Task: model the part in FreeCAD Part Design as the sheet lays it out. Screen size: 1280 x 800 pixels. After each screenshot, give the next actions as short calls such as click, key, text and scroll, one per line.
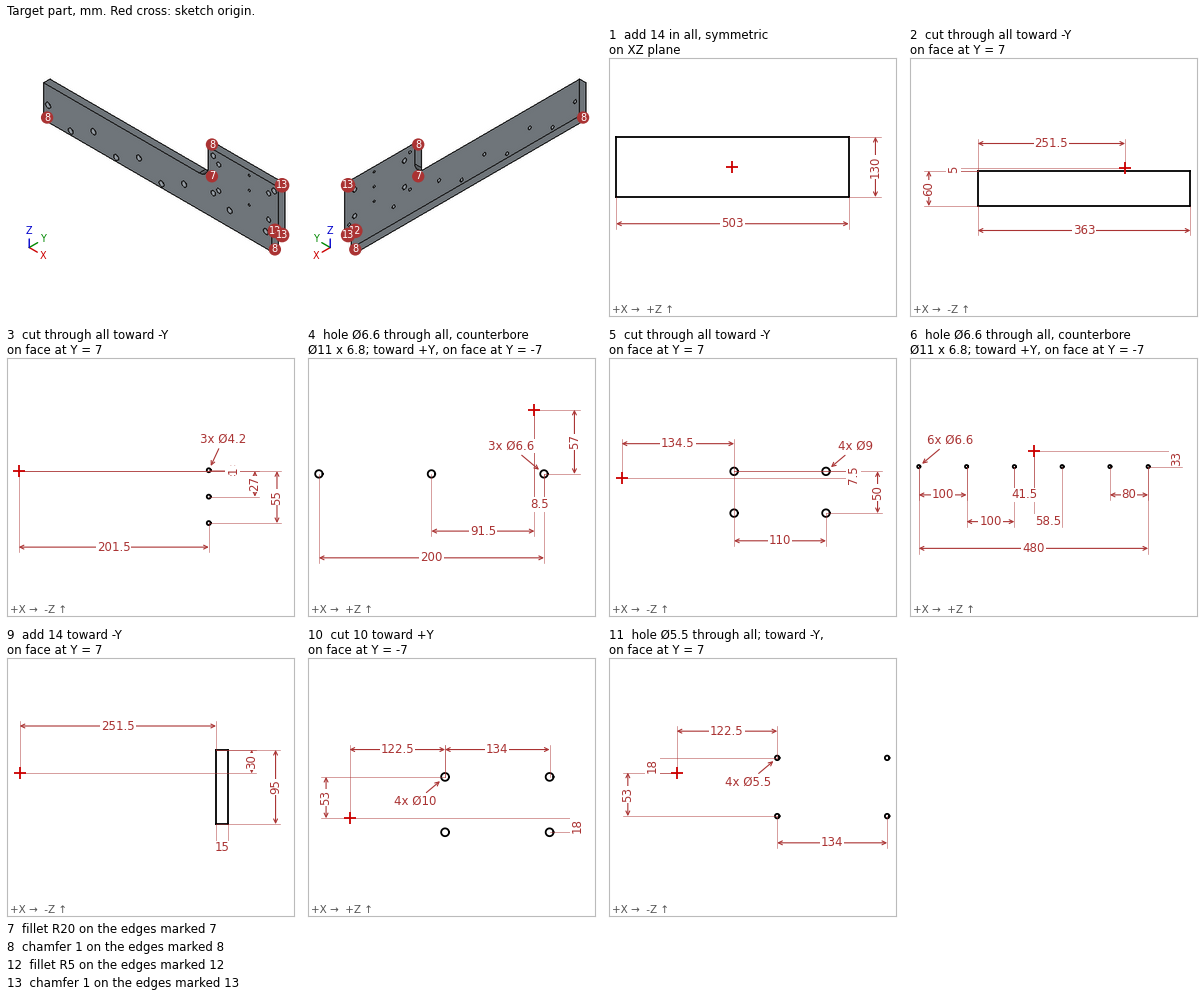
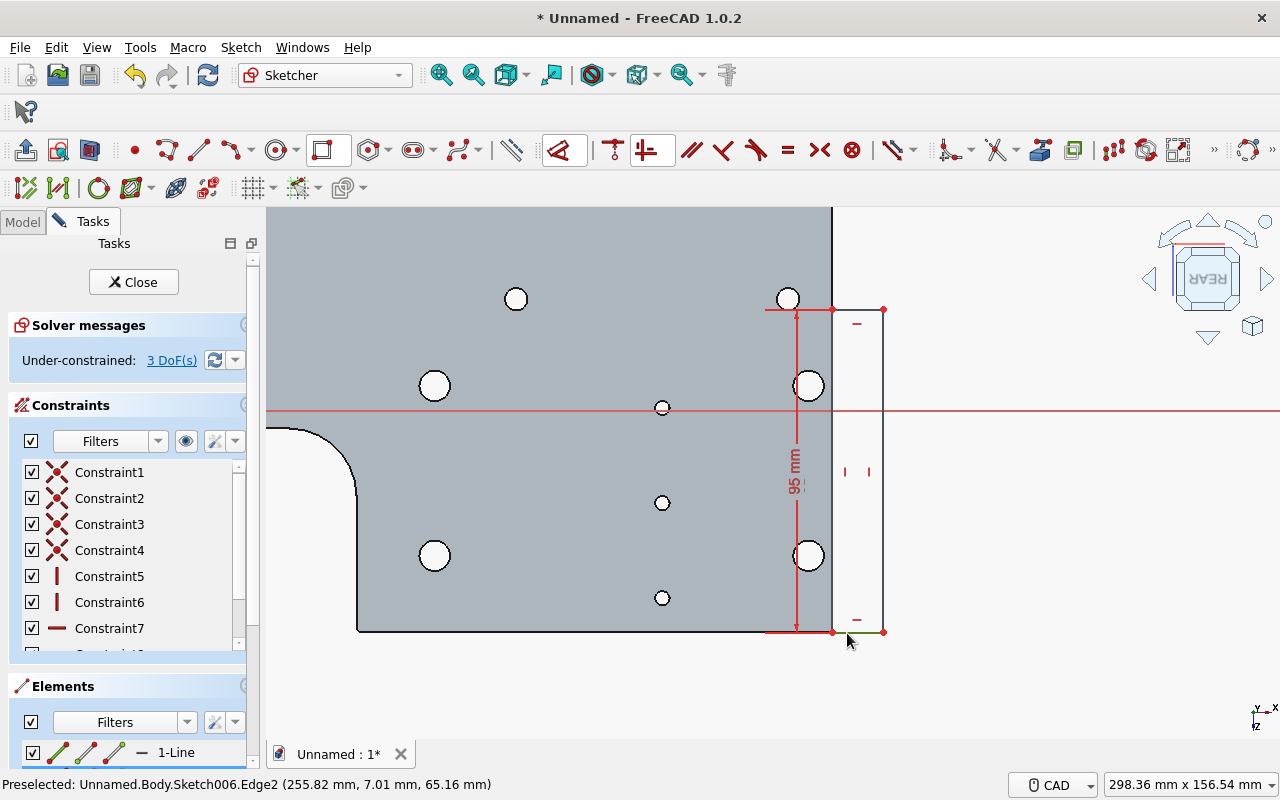
key(l)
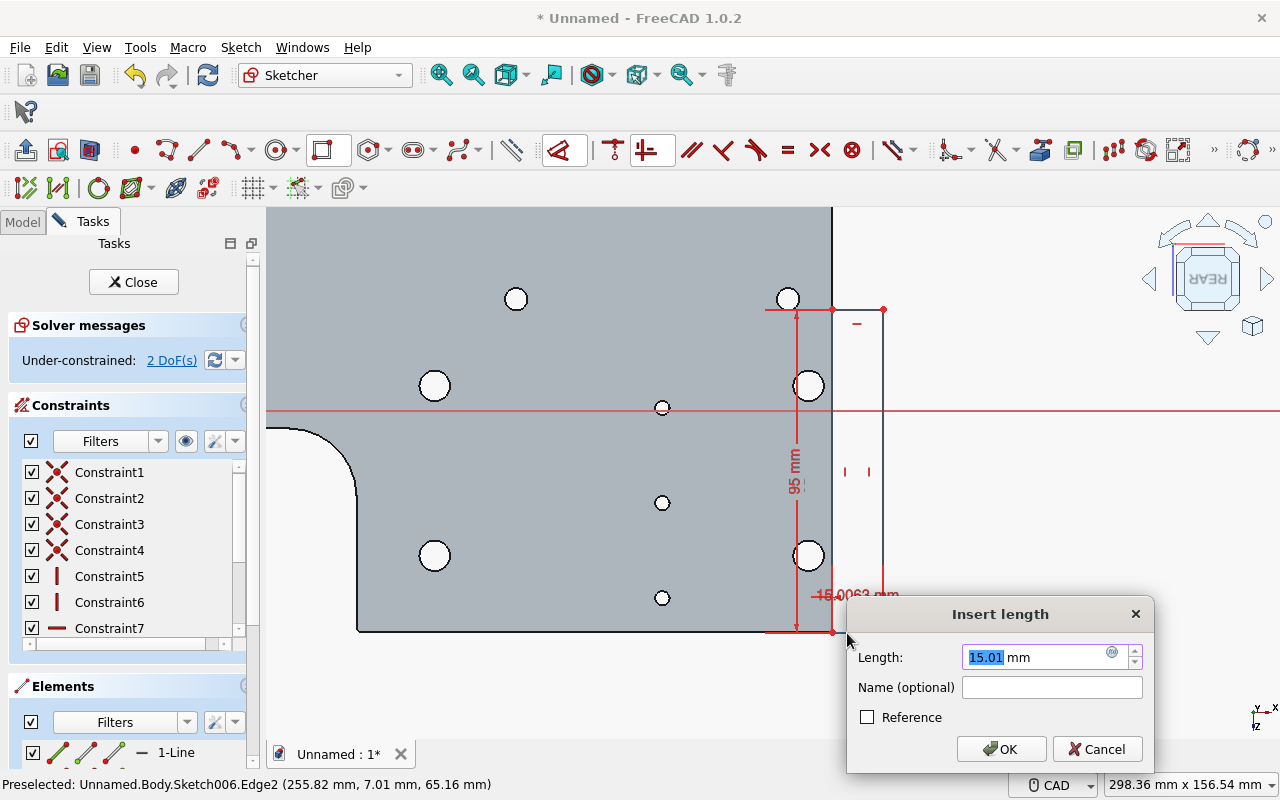
text(15)
key(Return)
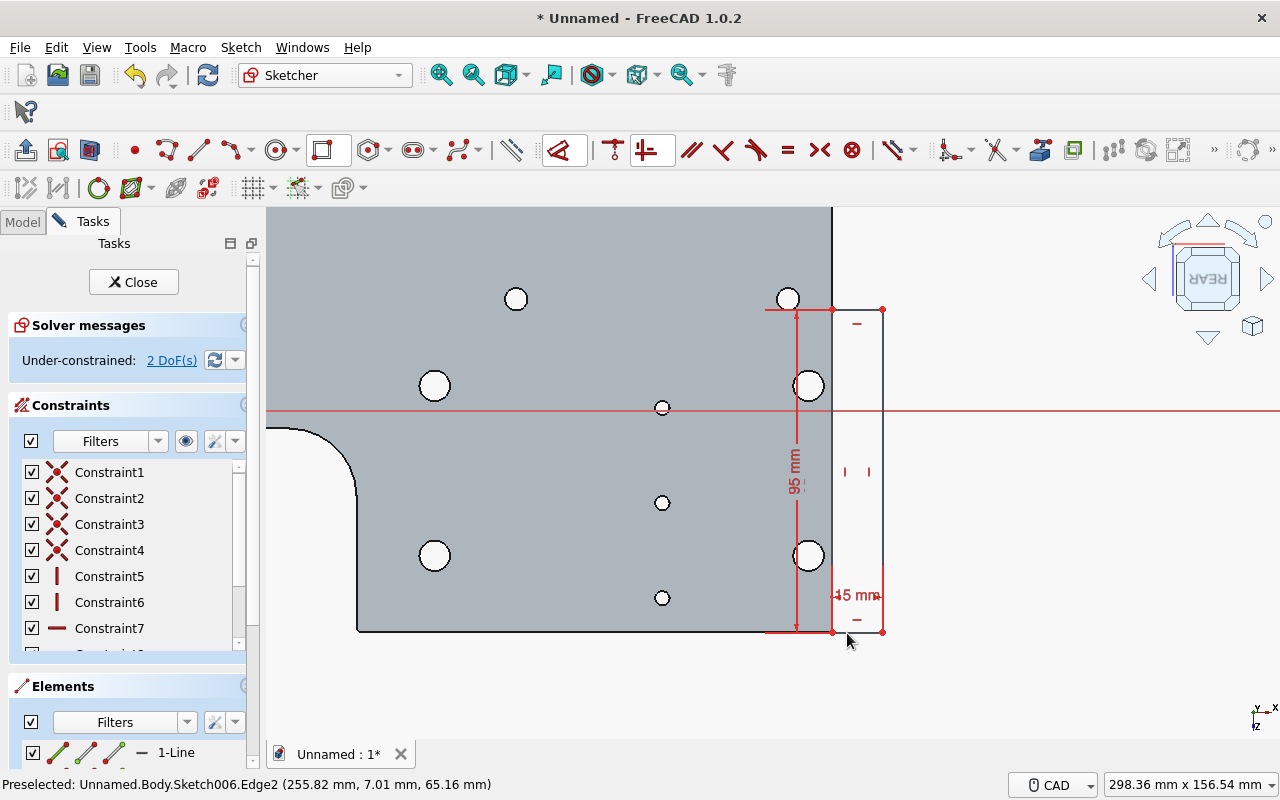
click(832, 310)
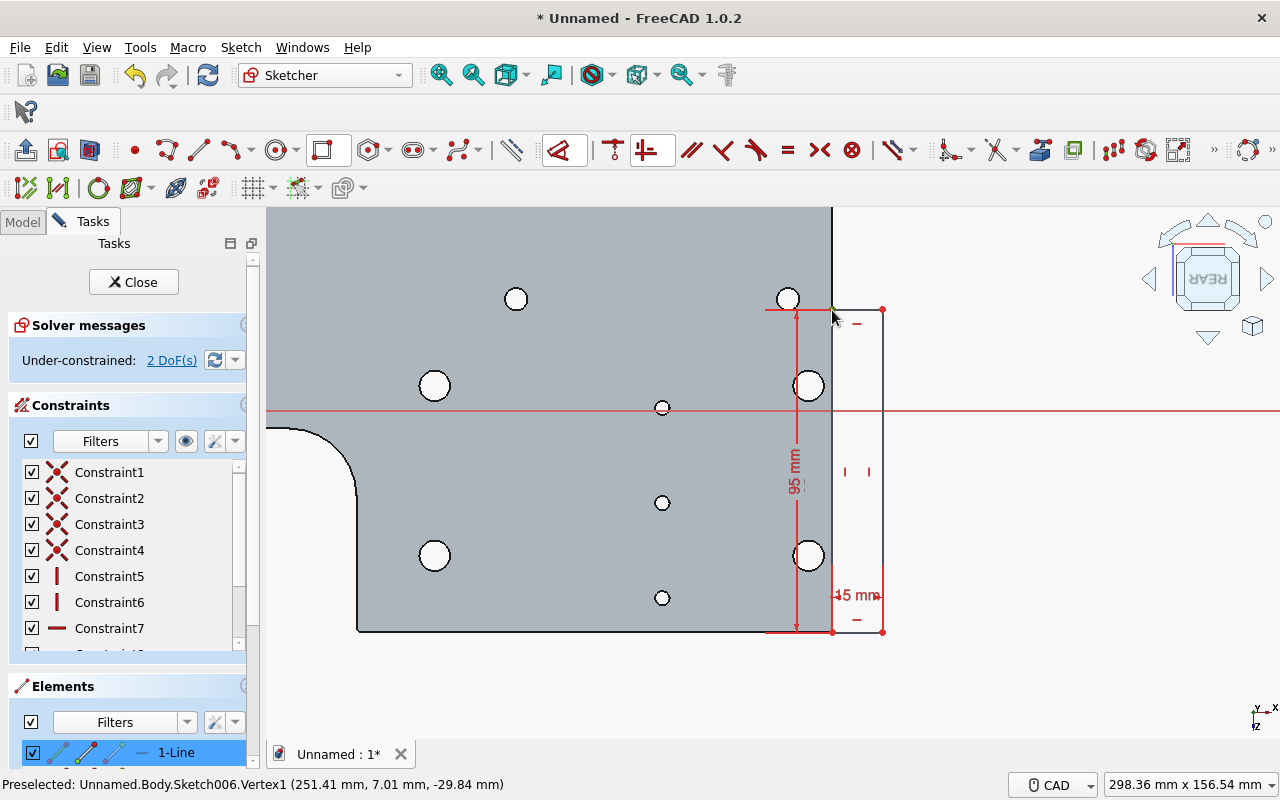
click(582, 150)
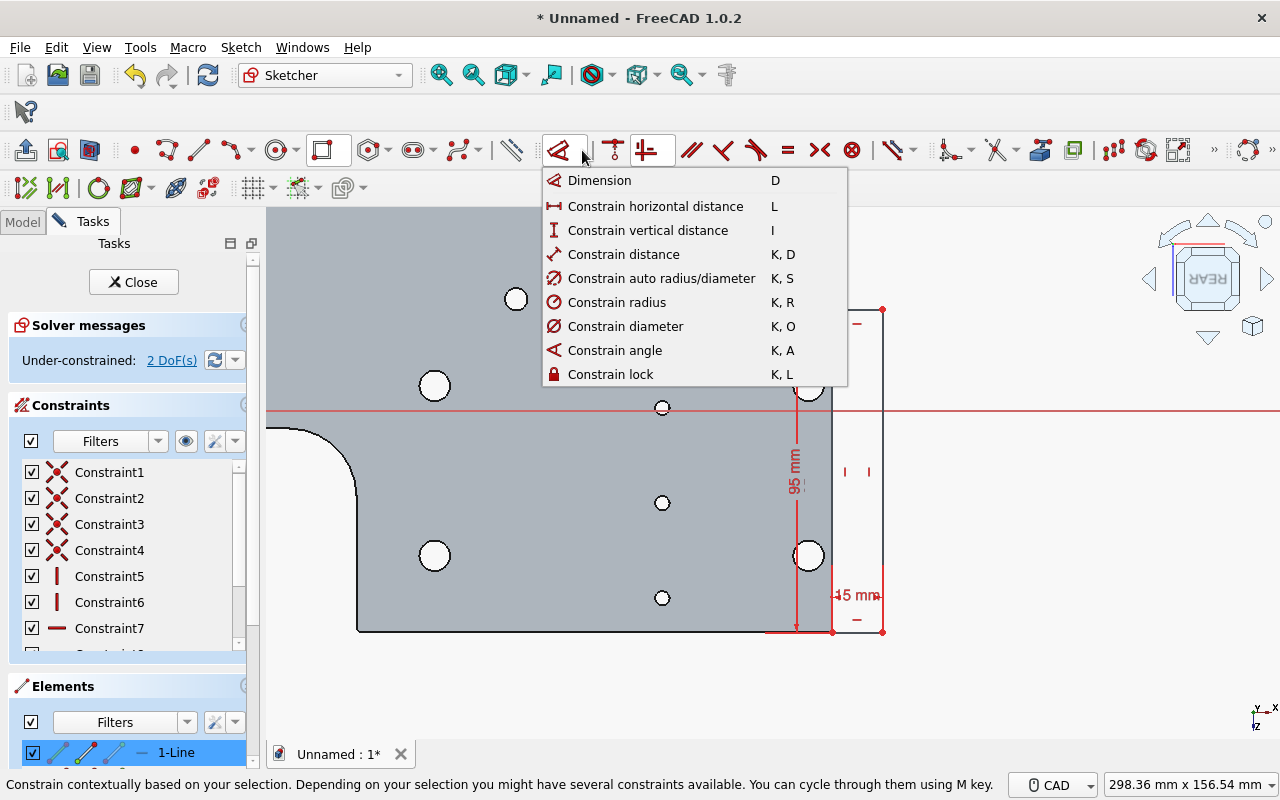
click(695, 230)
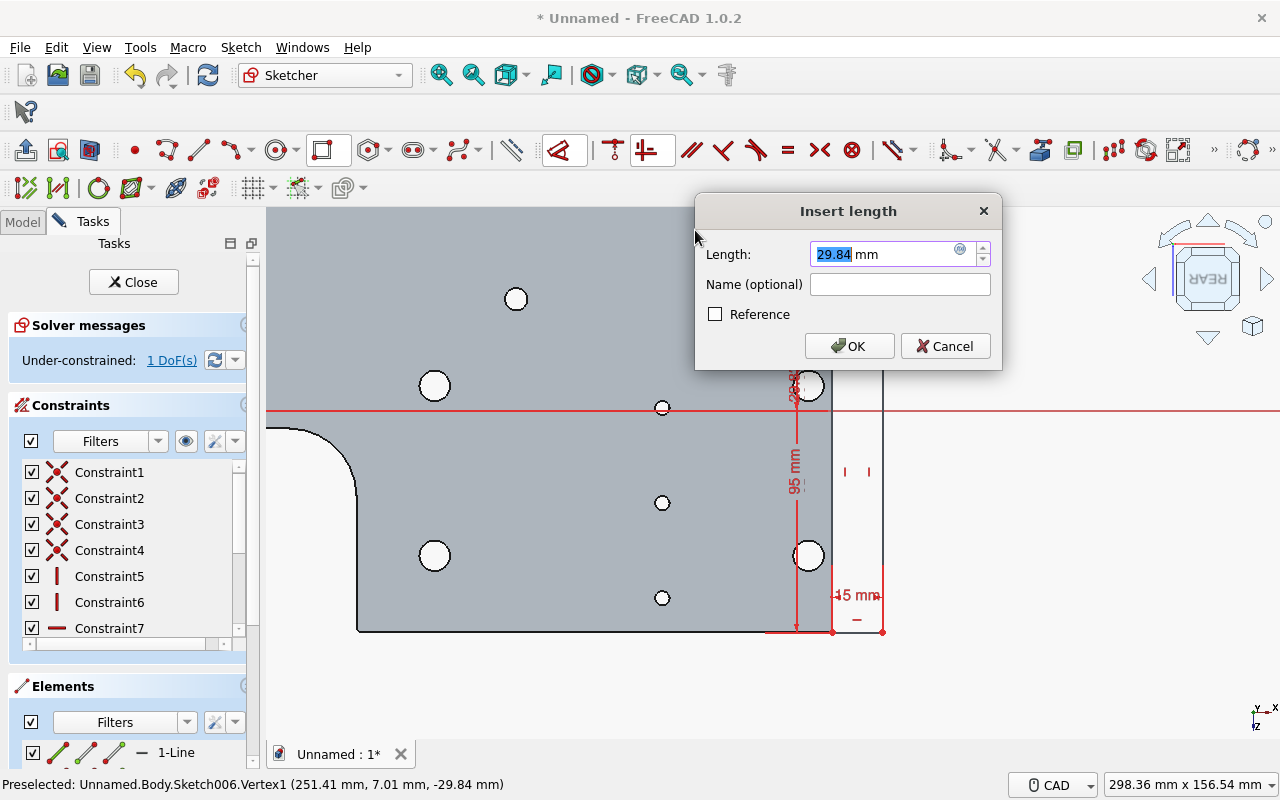
text(30)
key(Return)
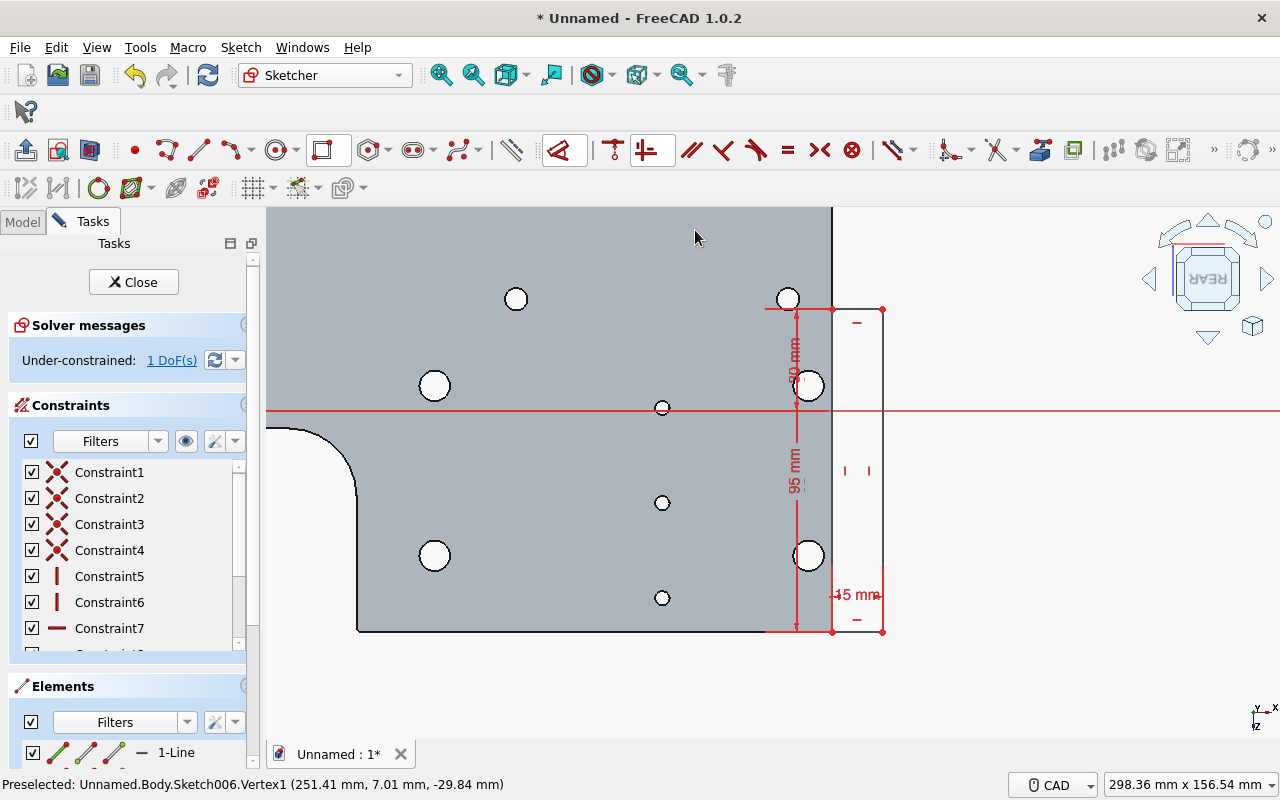
click(832, 309)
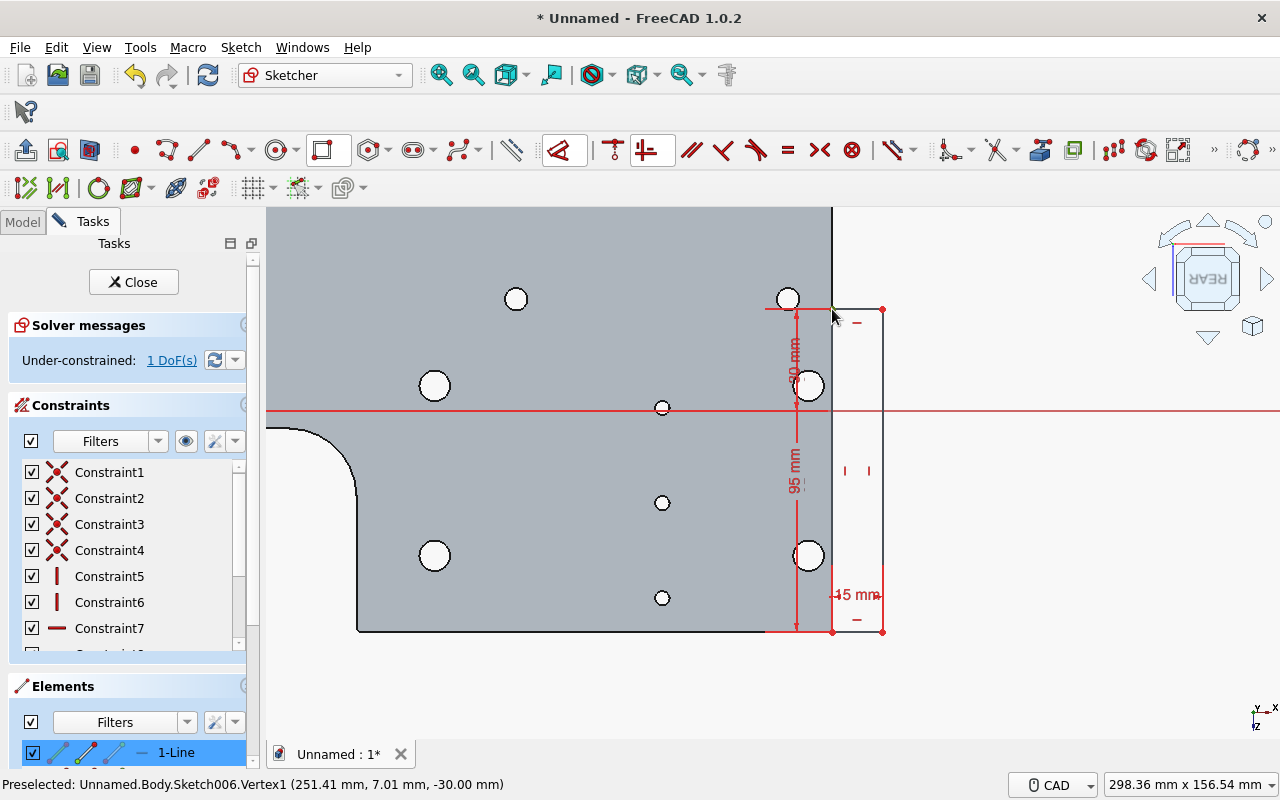
key(l)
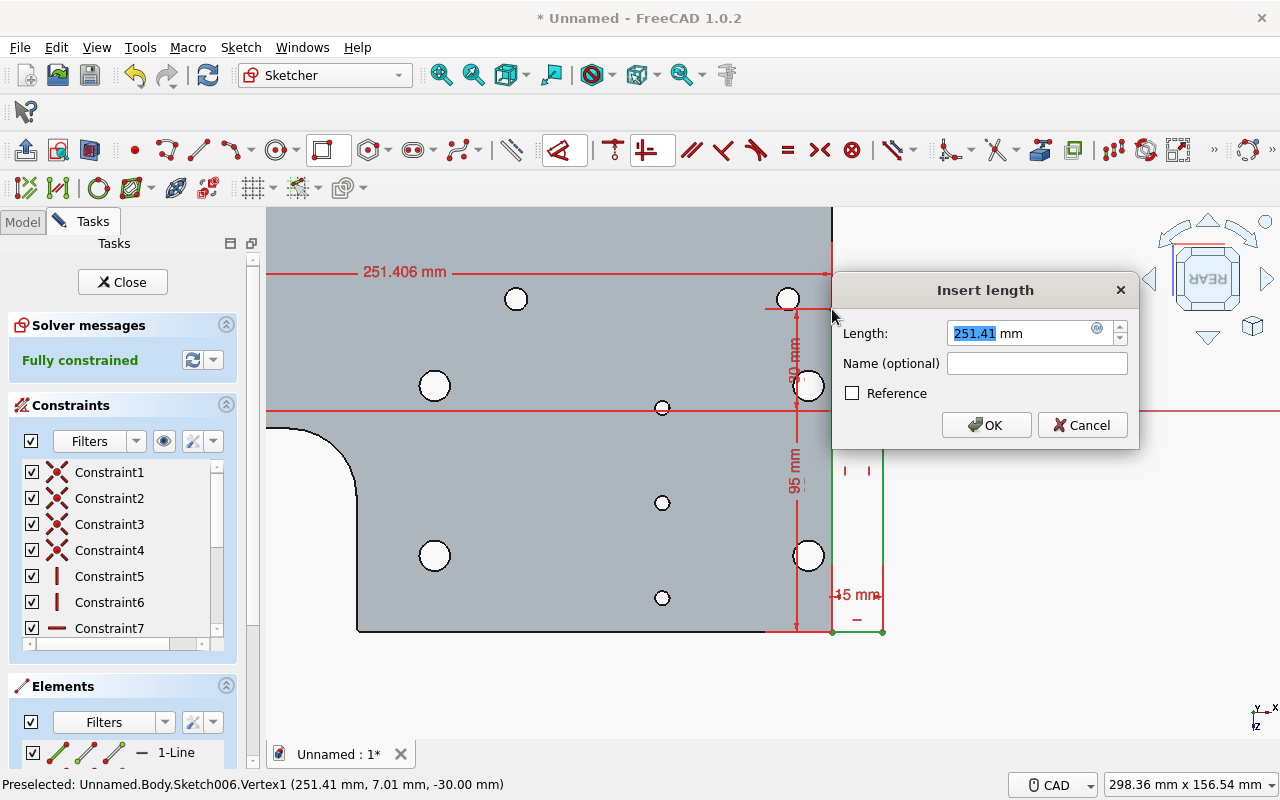
text(251.5)
key(Return)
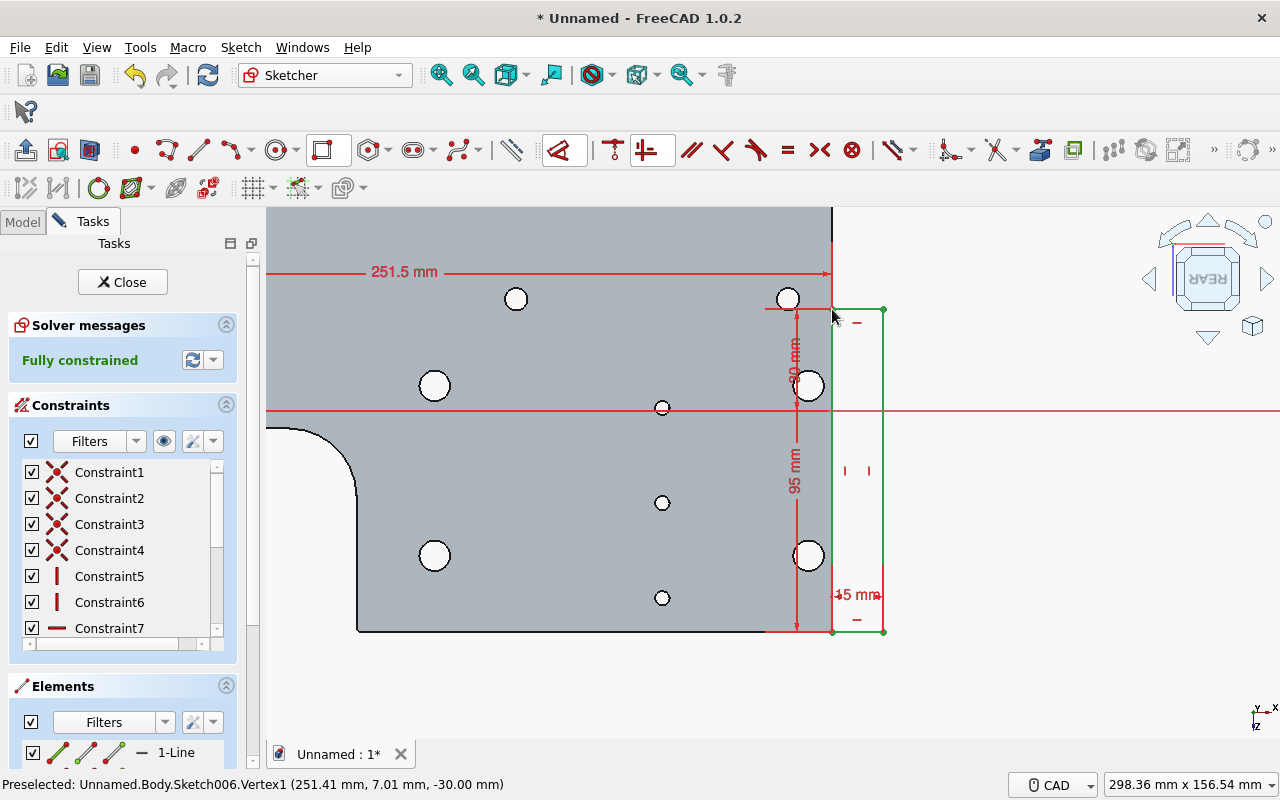
click(123, 282)